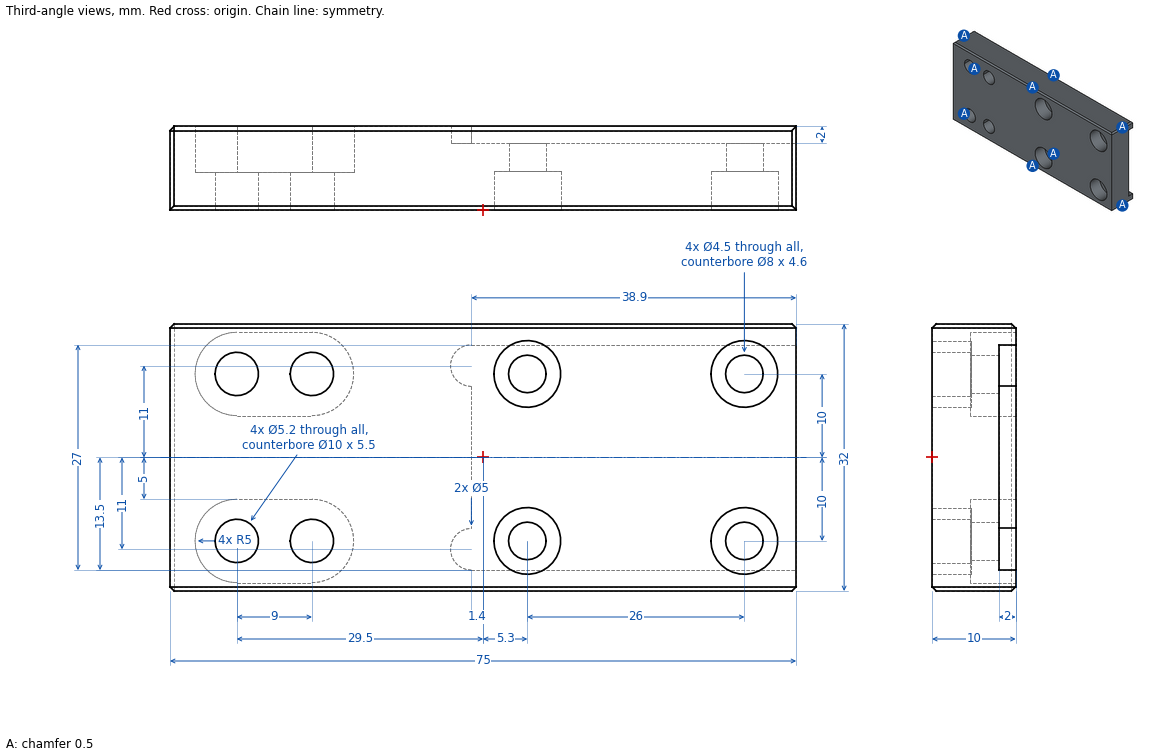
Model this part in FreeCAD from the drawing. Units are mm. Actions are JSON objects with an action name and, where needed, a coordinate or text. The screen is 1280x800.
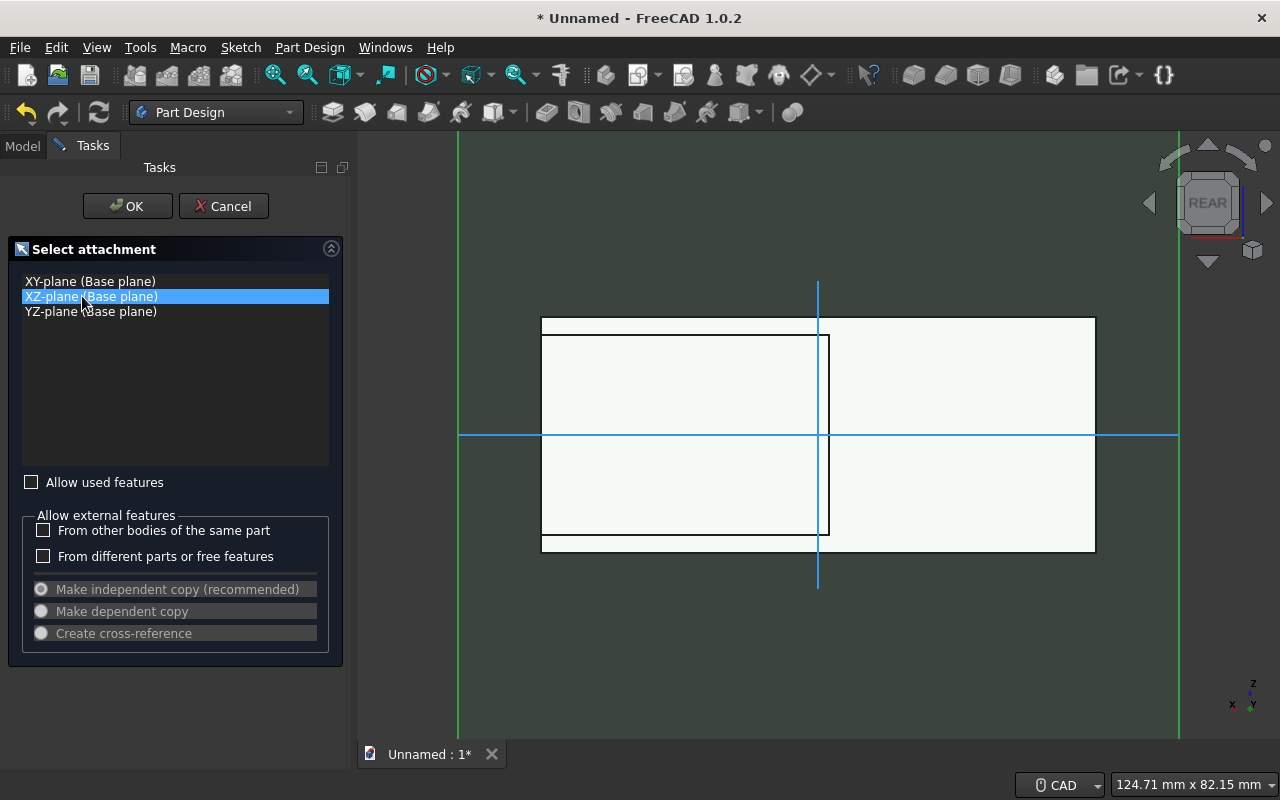
{"action": "left_click", "coordinate": [128, 206]}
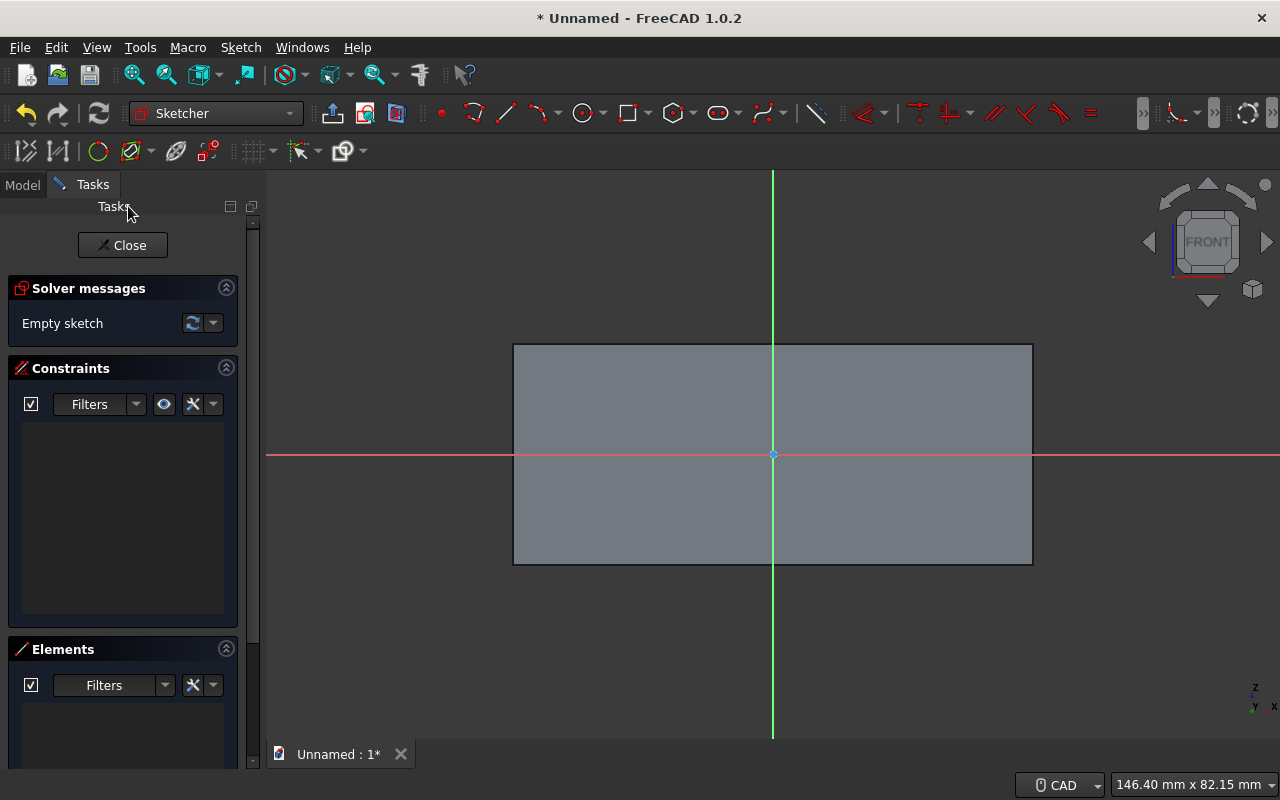
{"action": "scroll", "coordinate": [1040, 455], "scroll_direction": "up", "scroll_amount": 4}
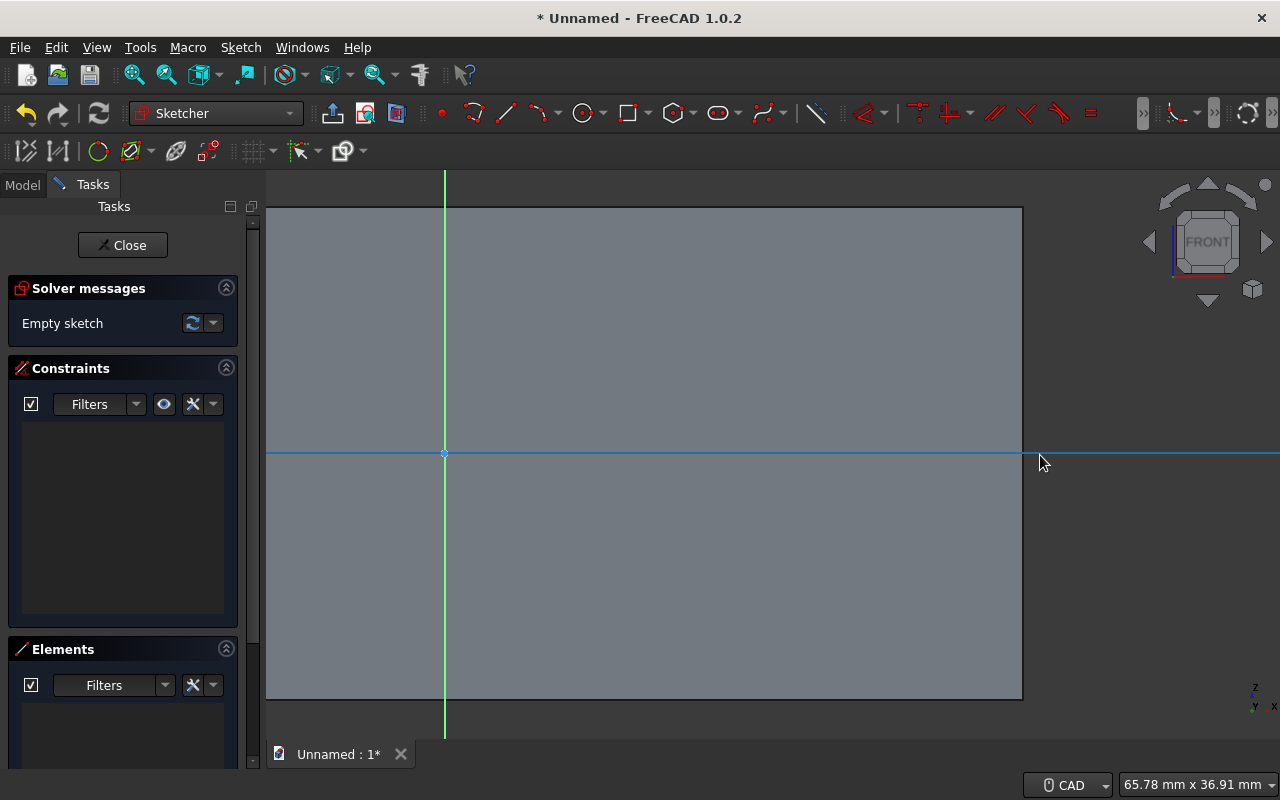
{"action": "left_click", "coordinate": [584, 114]}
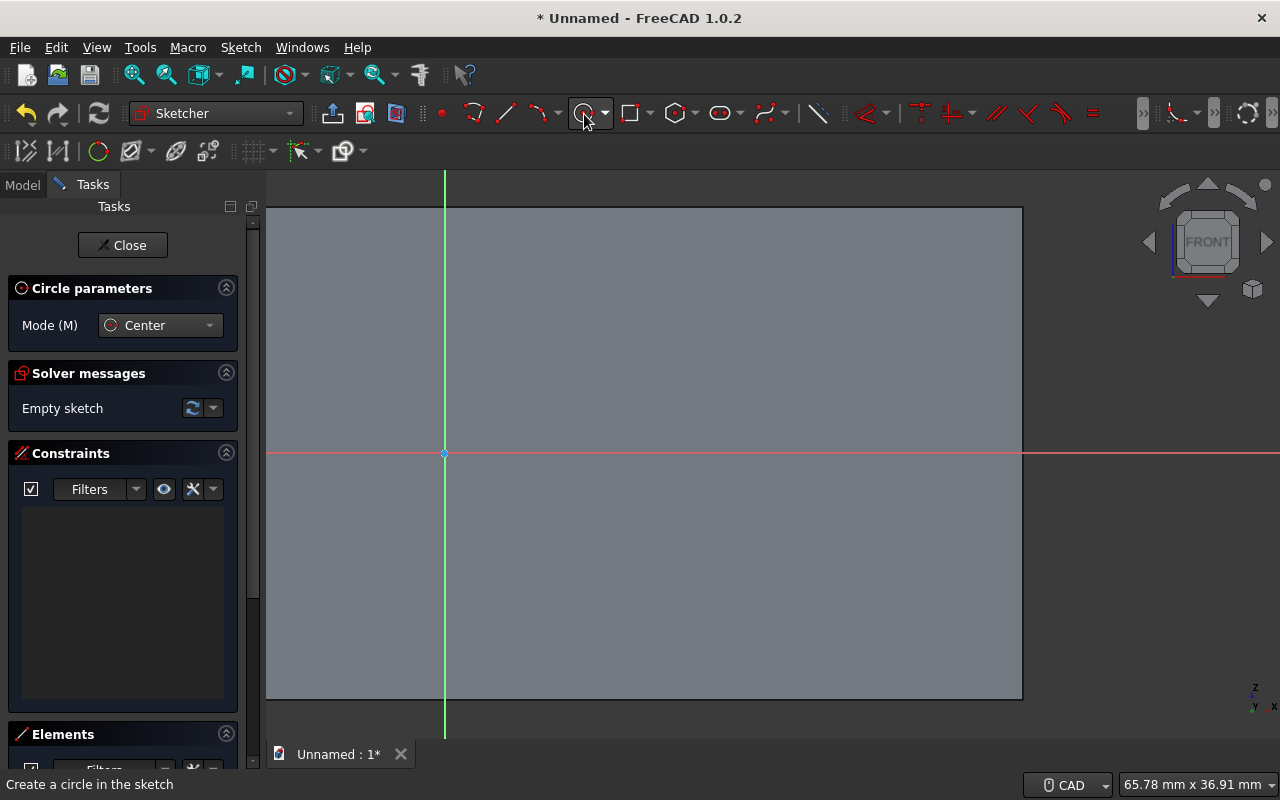
{"action": "left_click", "coordinate": [927, 299]}
{"action": "left_click", "coordinate": [952, 275]}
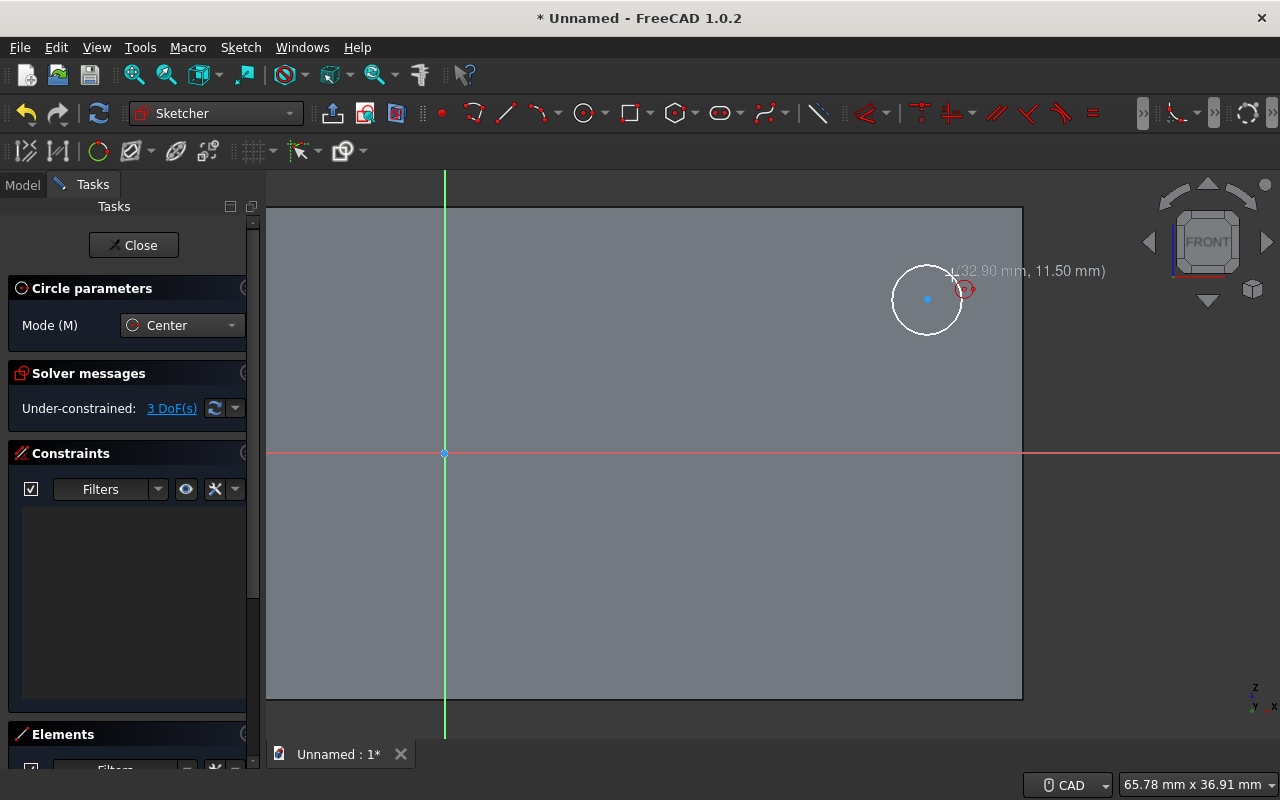
{"action": "left_click", "coordinate": [927, 607]}
{"action": "left_click", "coordinate": [952, 583]}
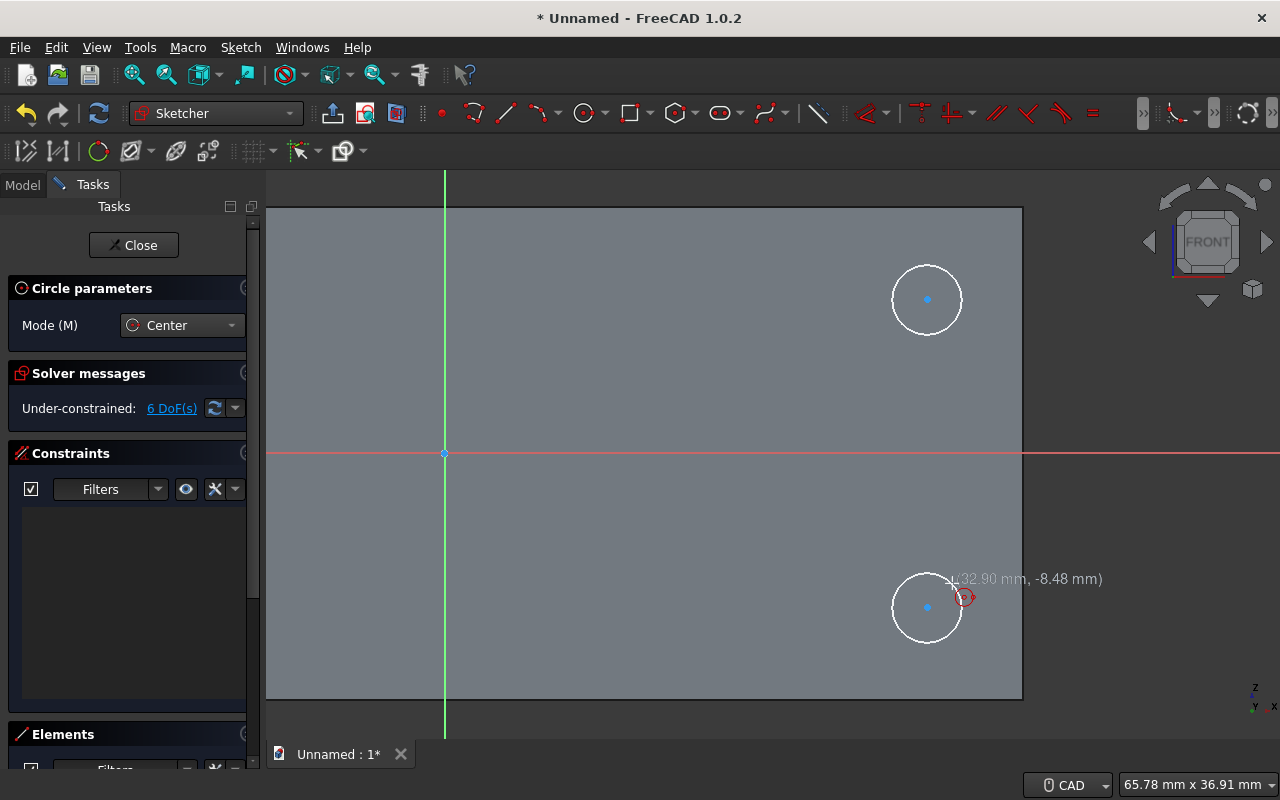
{"action": "left_click", "coordinate": [527, 607]}
{"action": "left_click", "coordinate": [551, 583]}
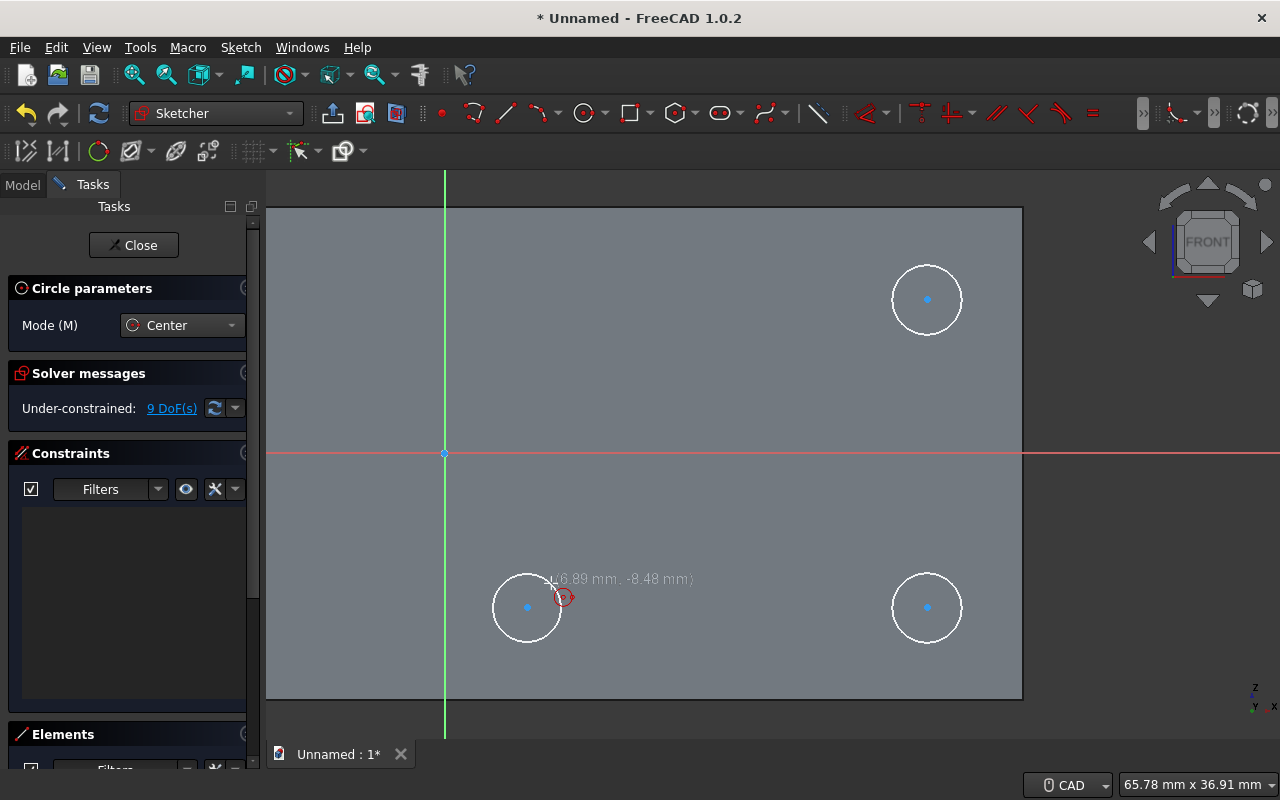
{"action": "left_click", "coordinate": [527, 299]}
{"action": "left_click", "coordinate": [551, 275]}
{"action": "key", "text": "Escape"}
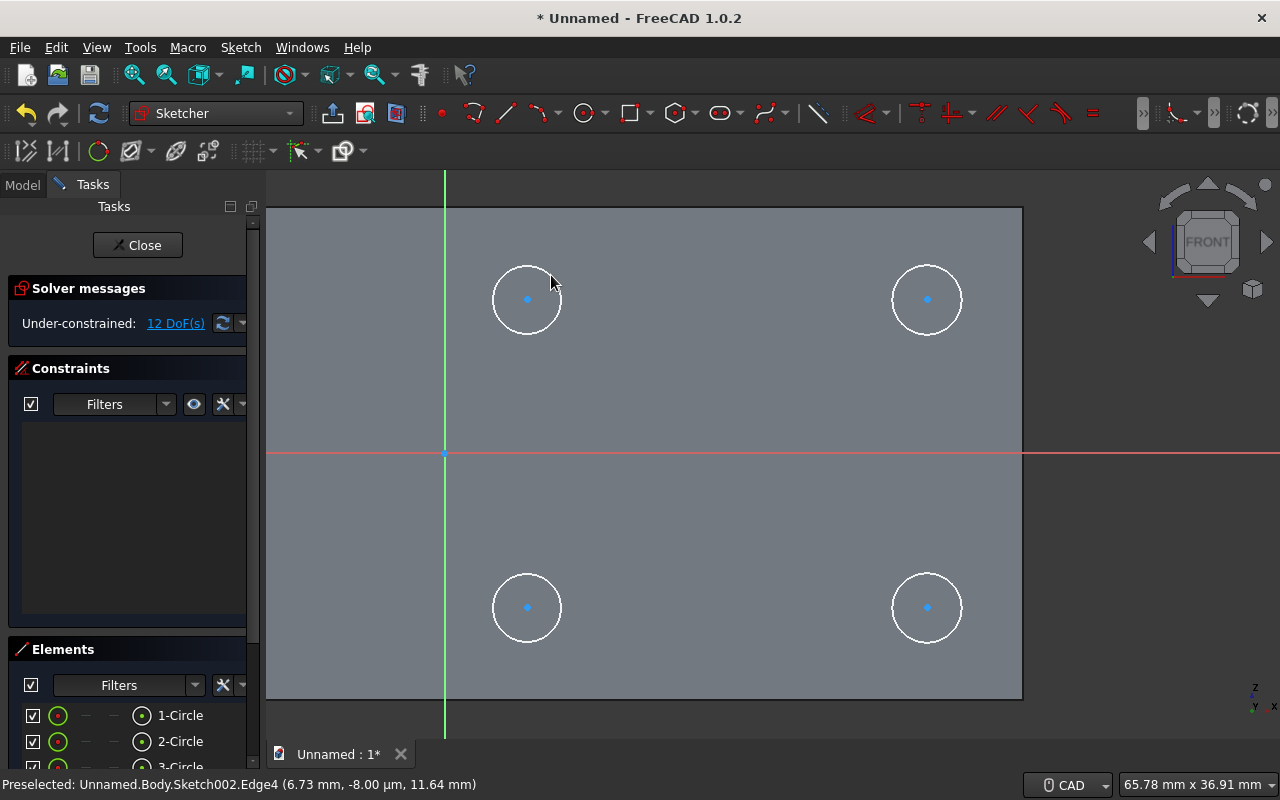
{"action": "left_click", "coordinate": [951, 275]}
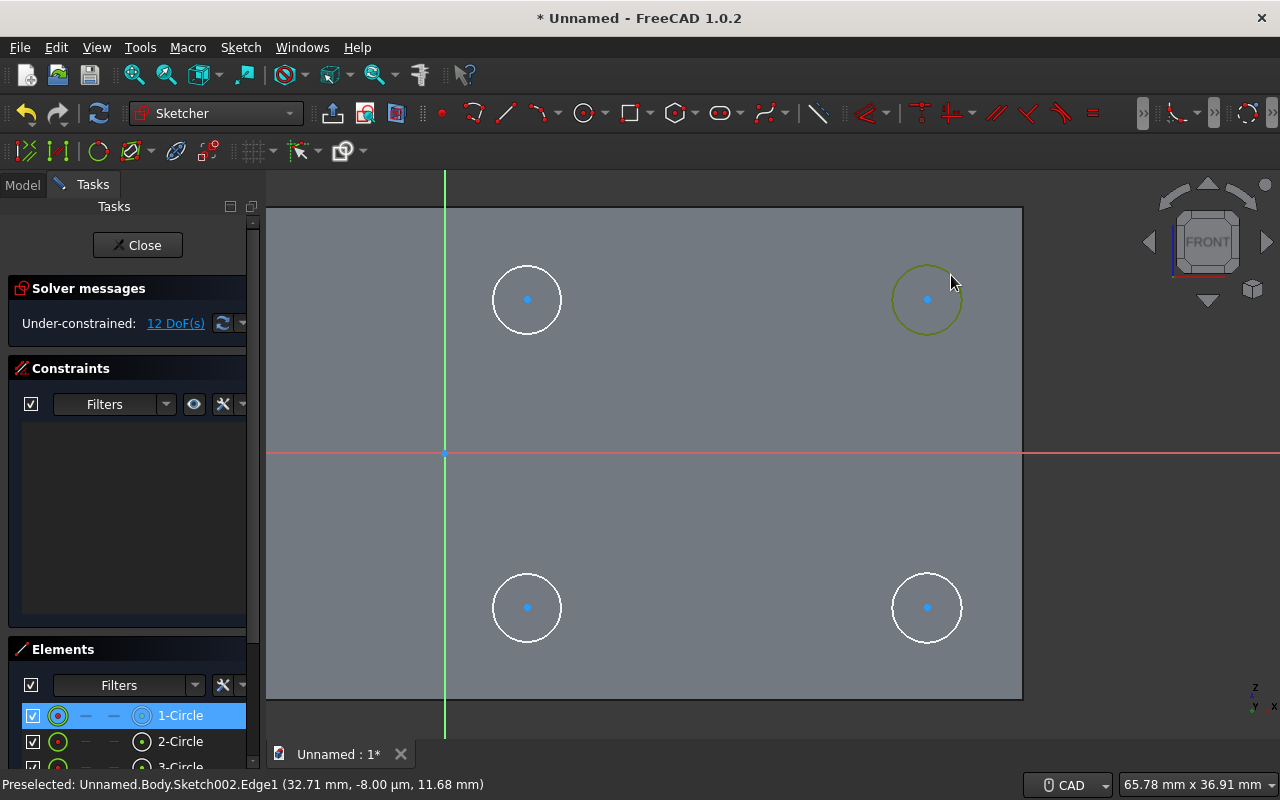
{"action": "left_click", "coordinate": [951, 583]}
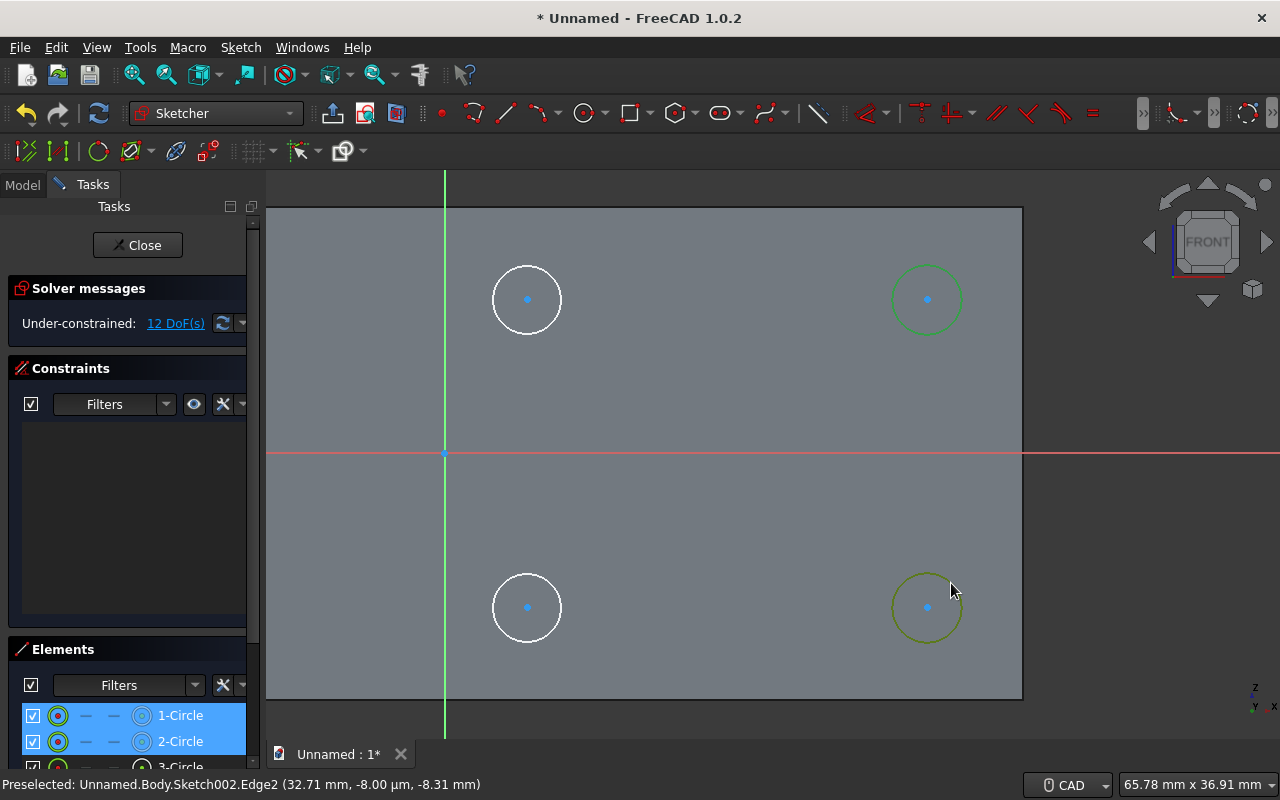
{"action": "left_click", "coordinate": [551, 584]}